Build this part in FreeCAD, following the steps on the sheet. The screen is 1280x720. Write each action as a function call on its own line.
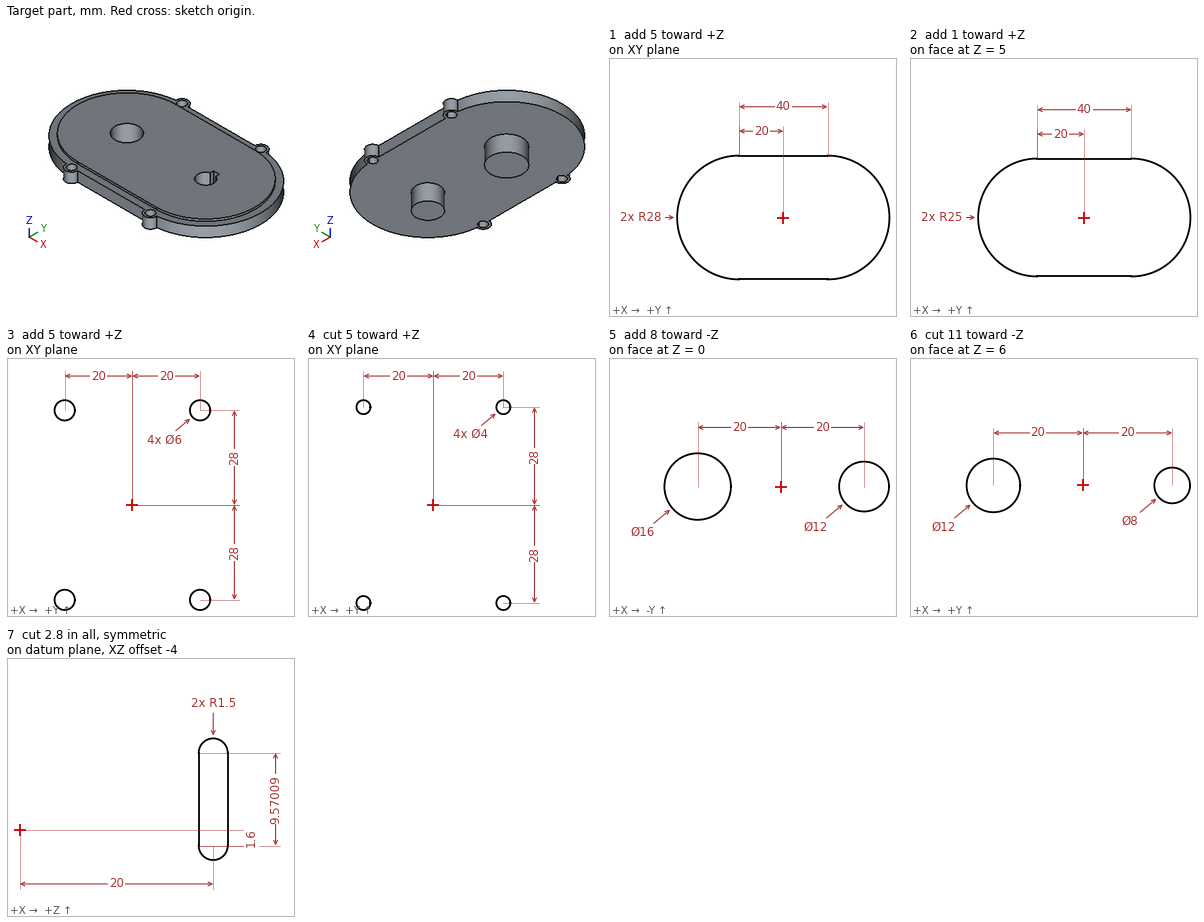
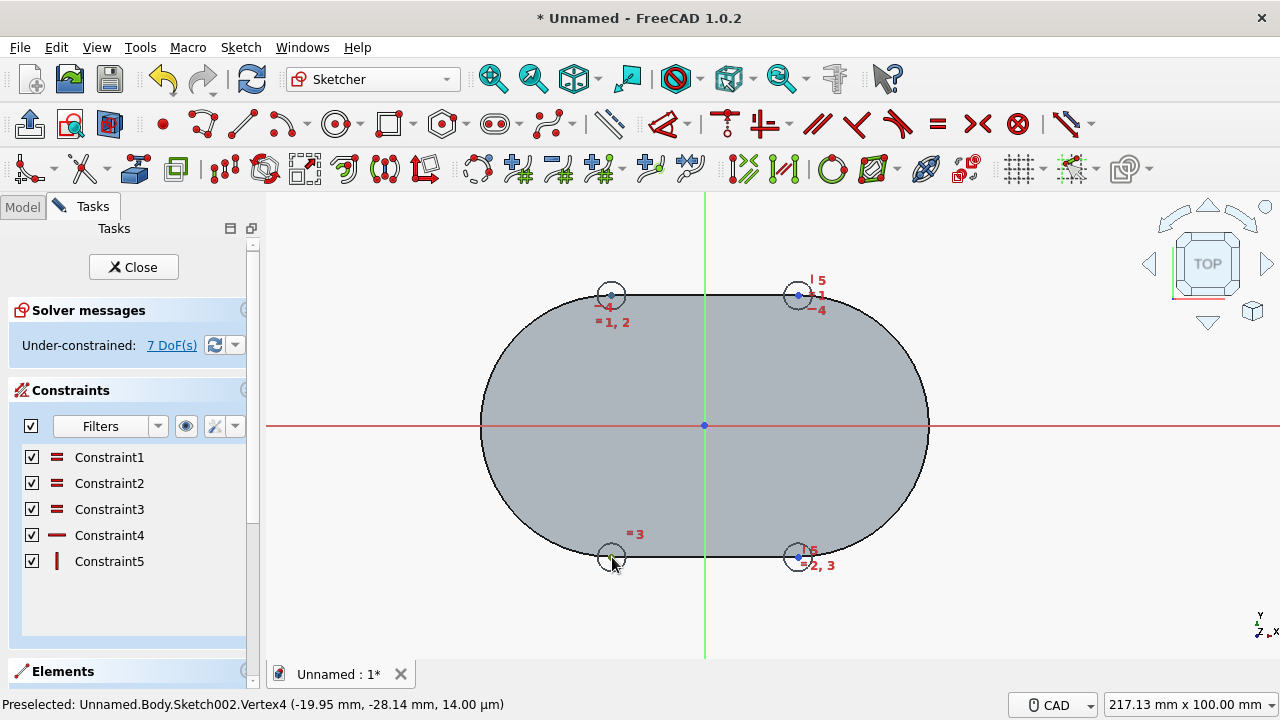
key(v)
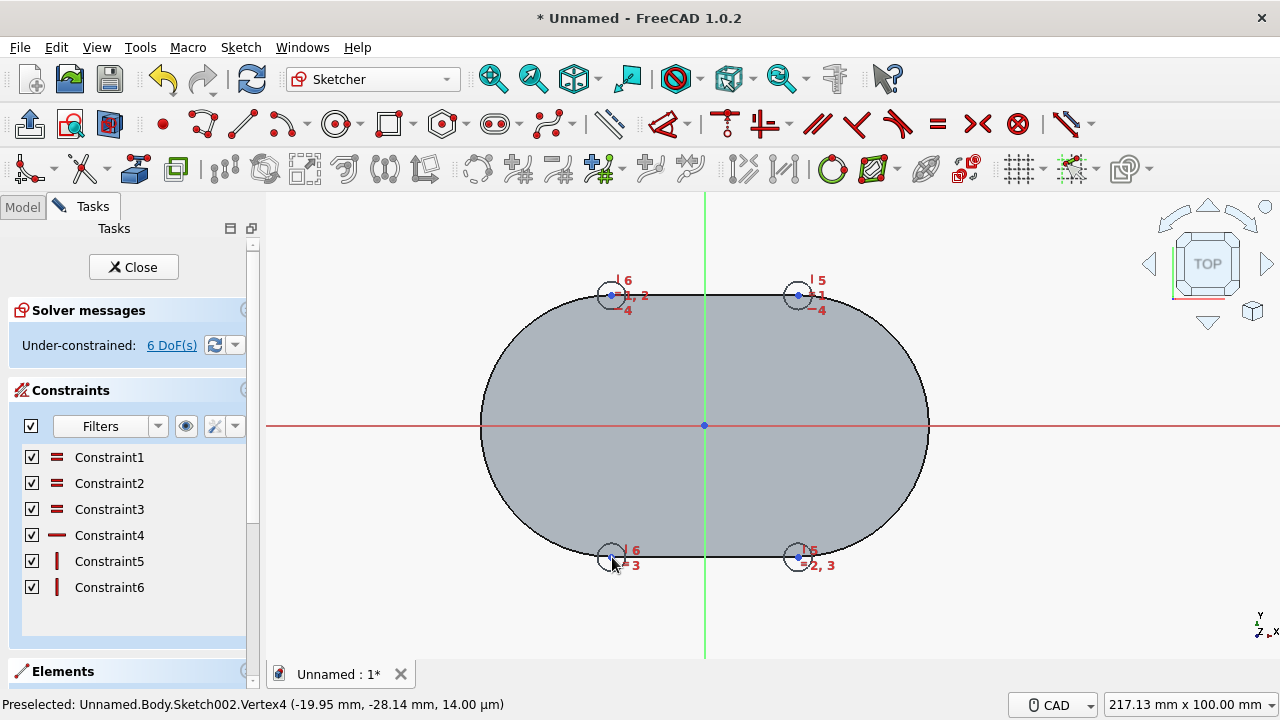
click(798, 557)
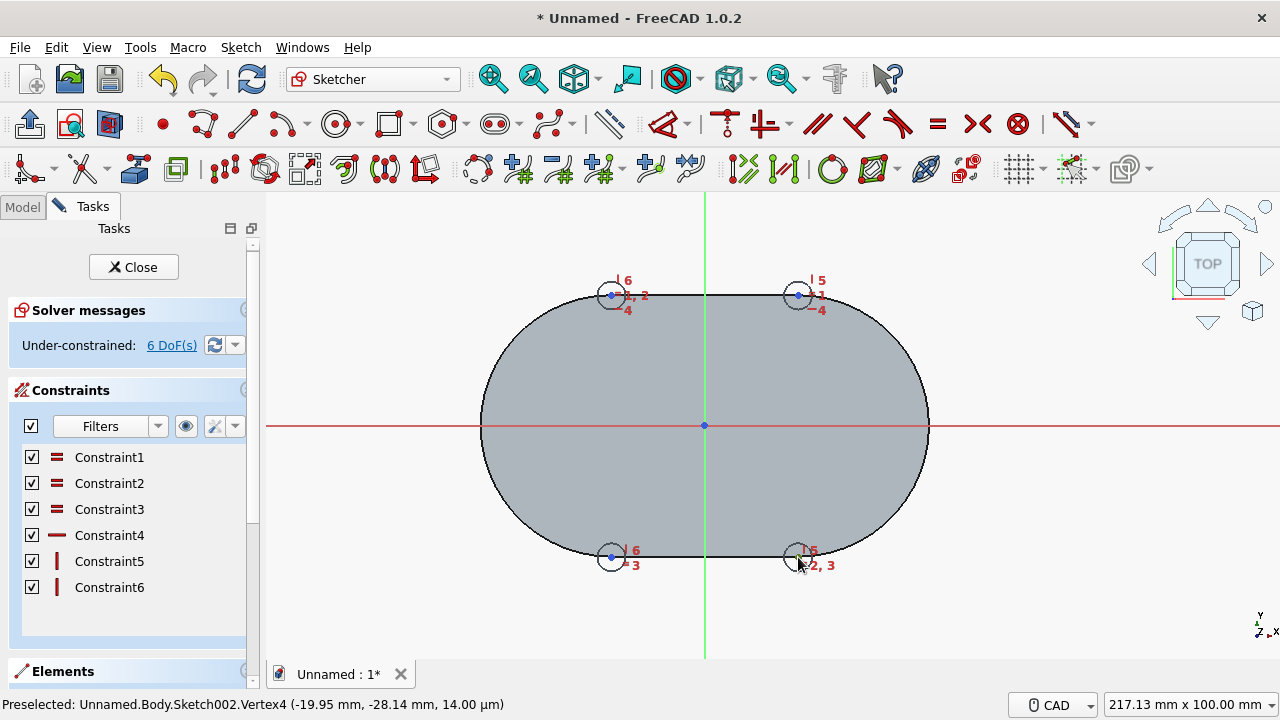
click(611, 557)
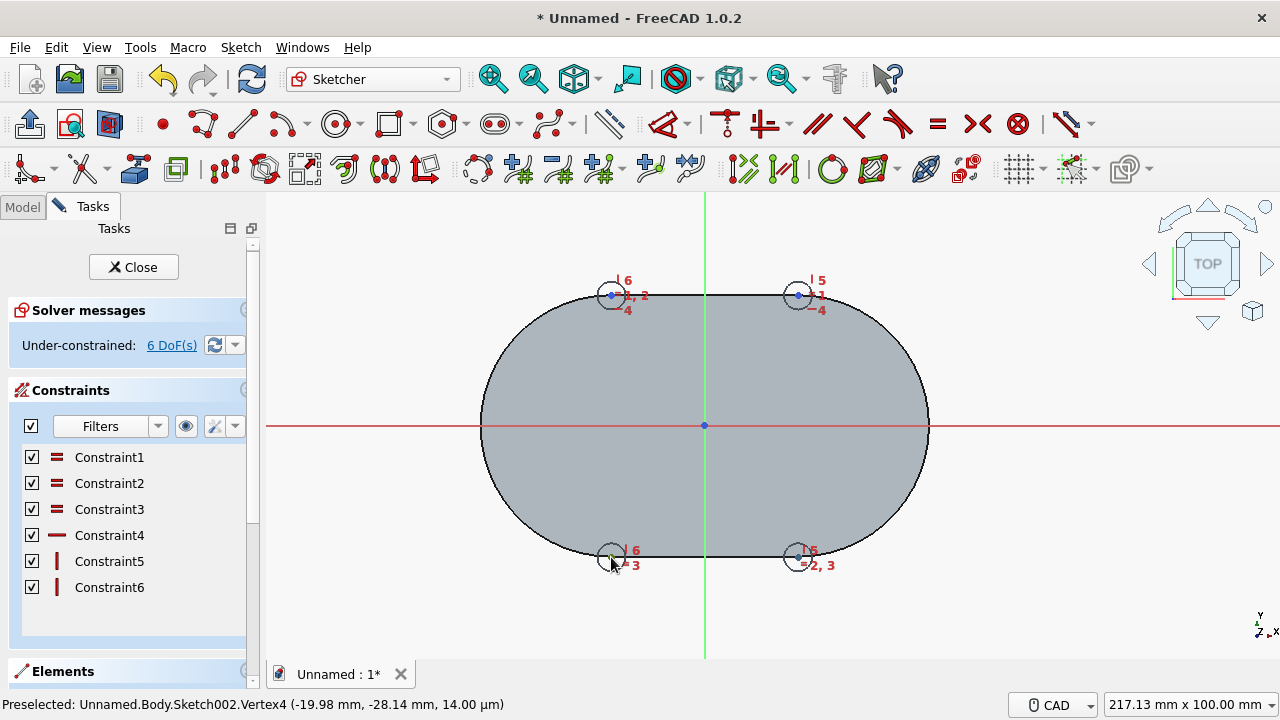
key(h)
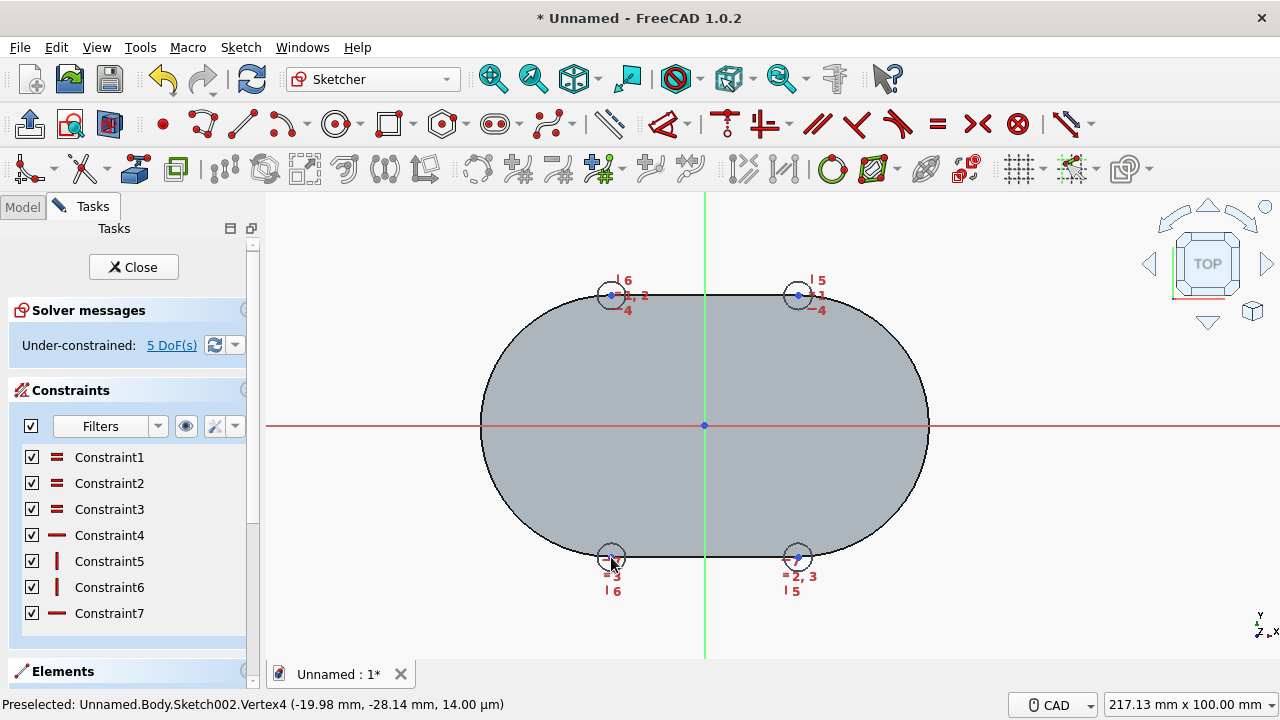
key(d)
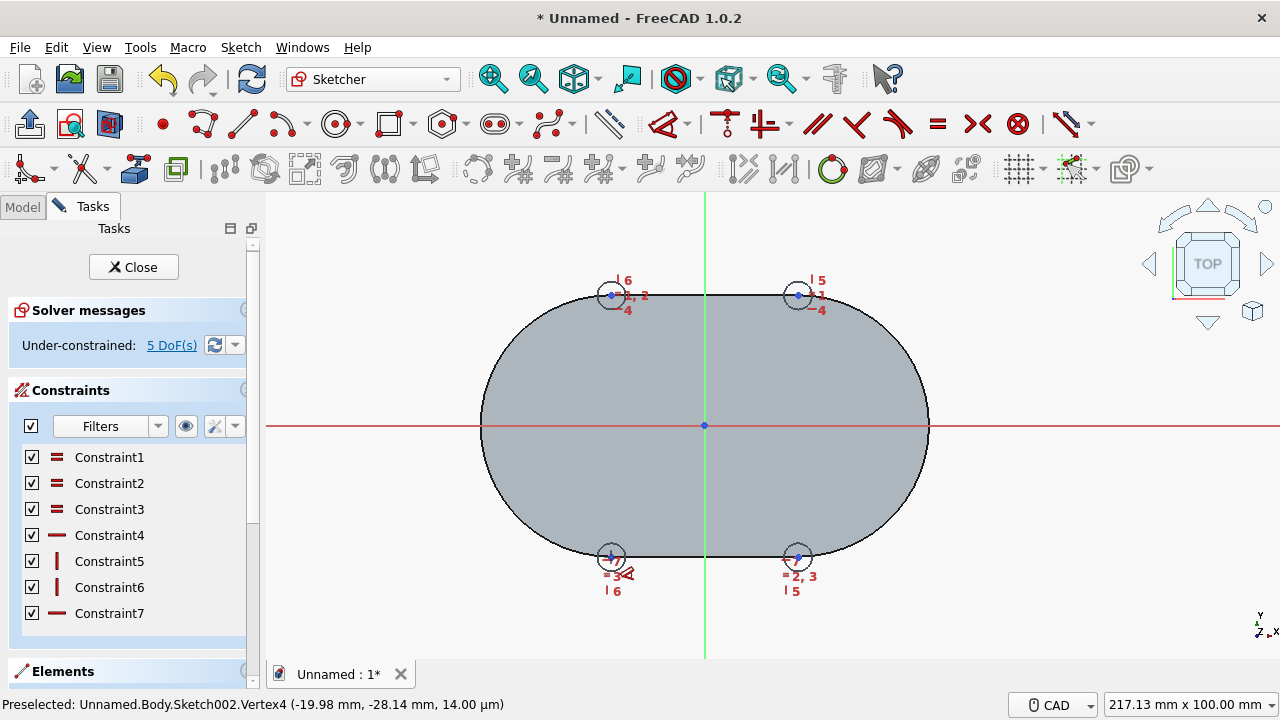
scroll(808, 286, up, 2)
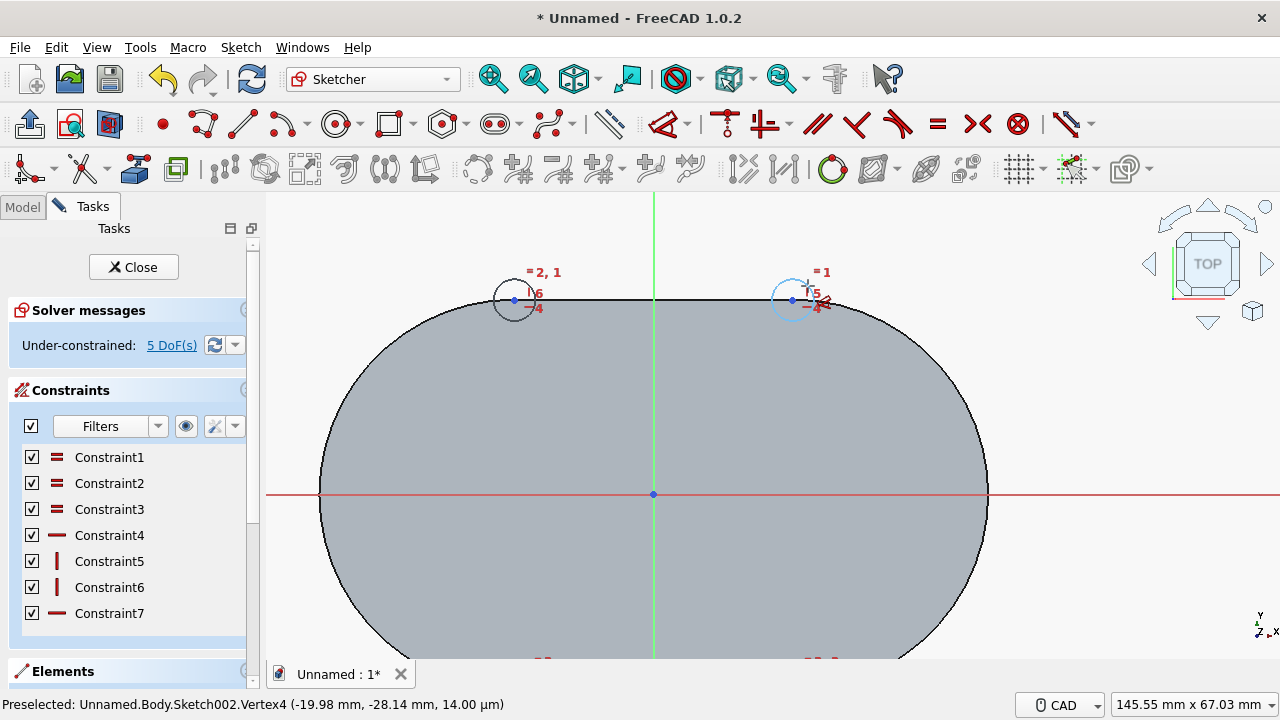
click(808, 285)
click(831, 262)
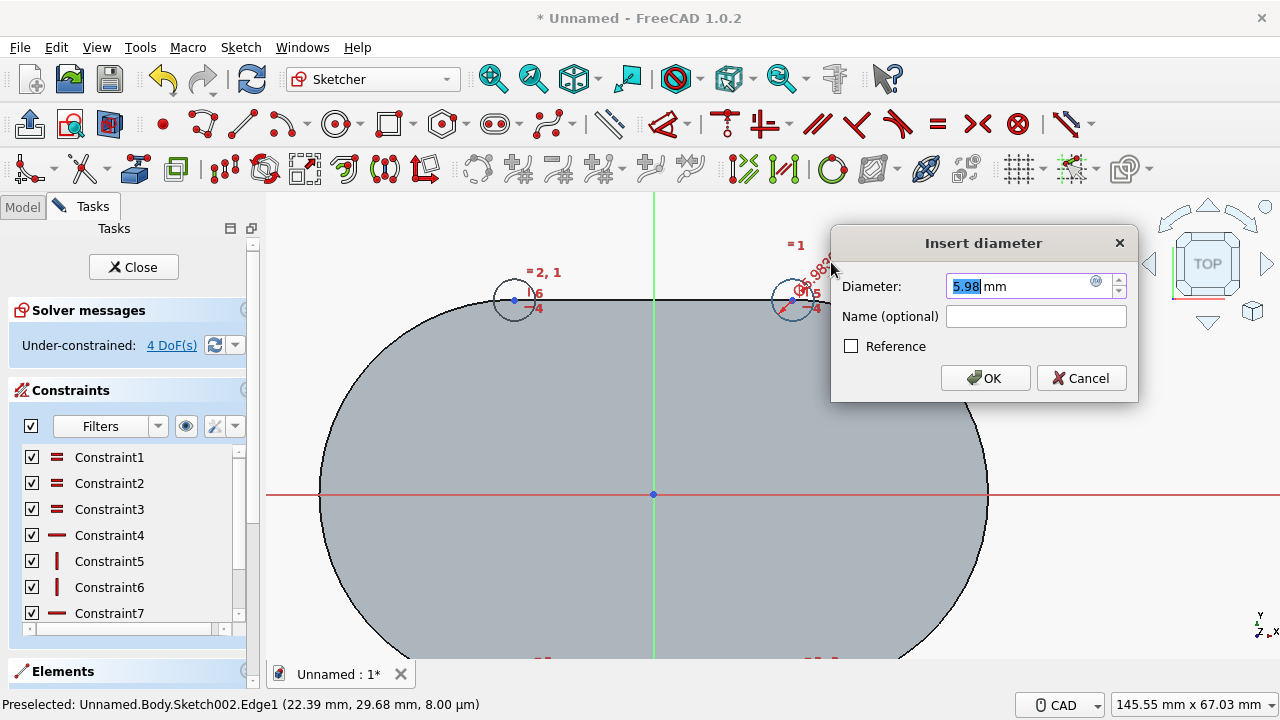
text(6)
key(Return)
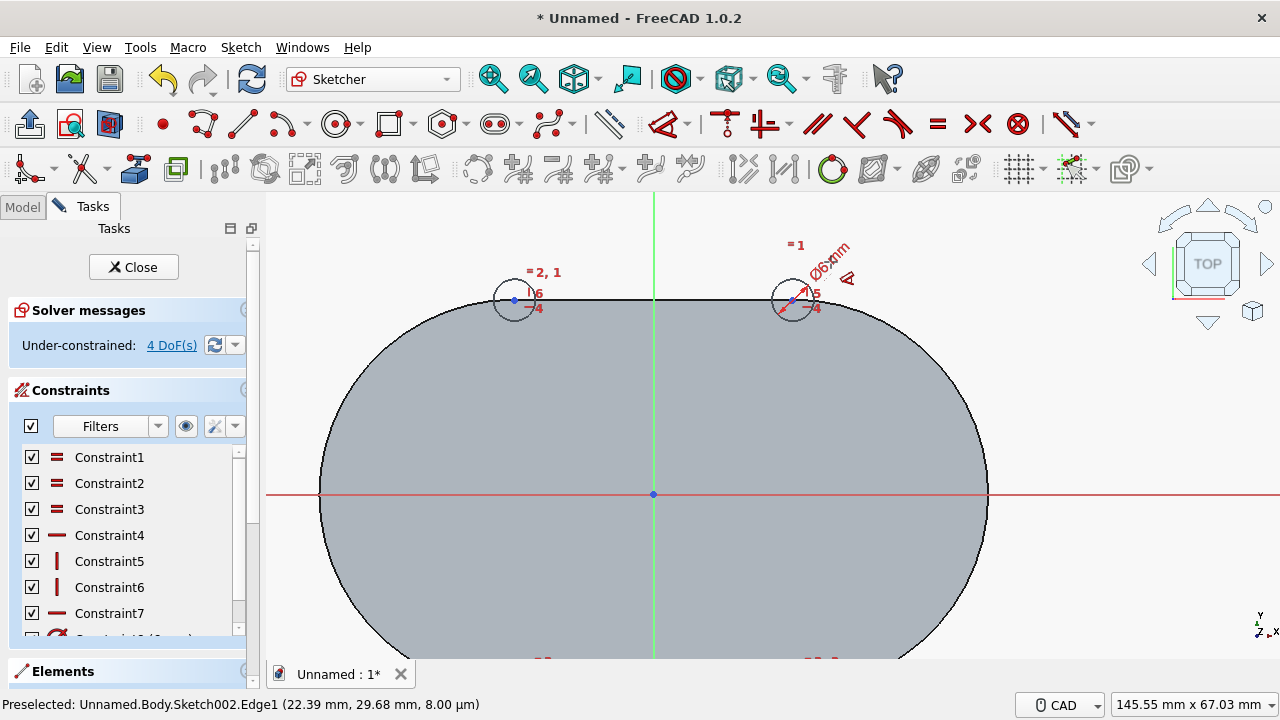
click(793, 300)
click(723, 266)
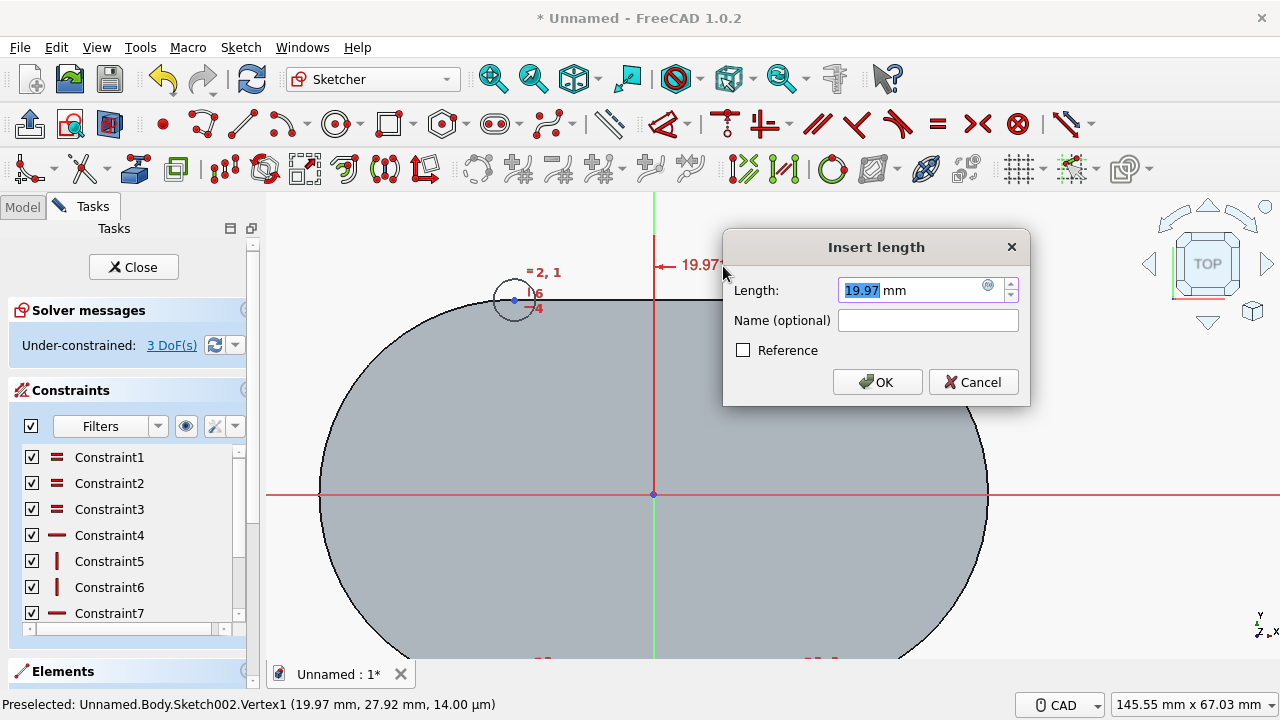
text(20)
key(Return)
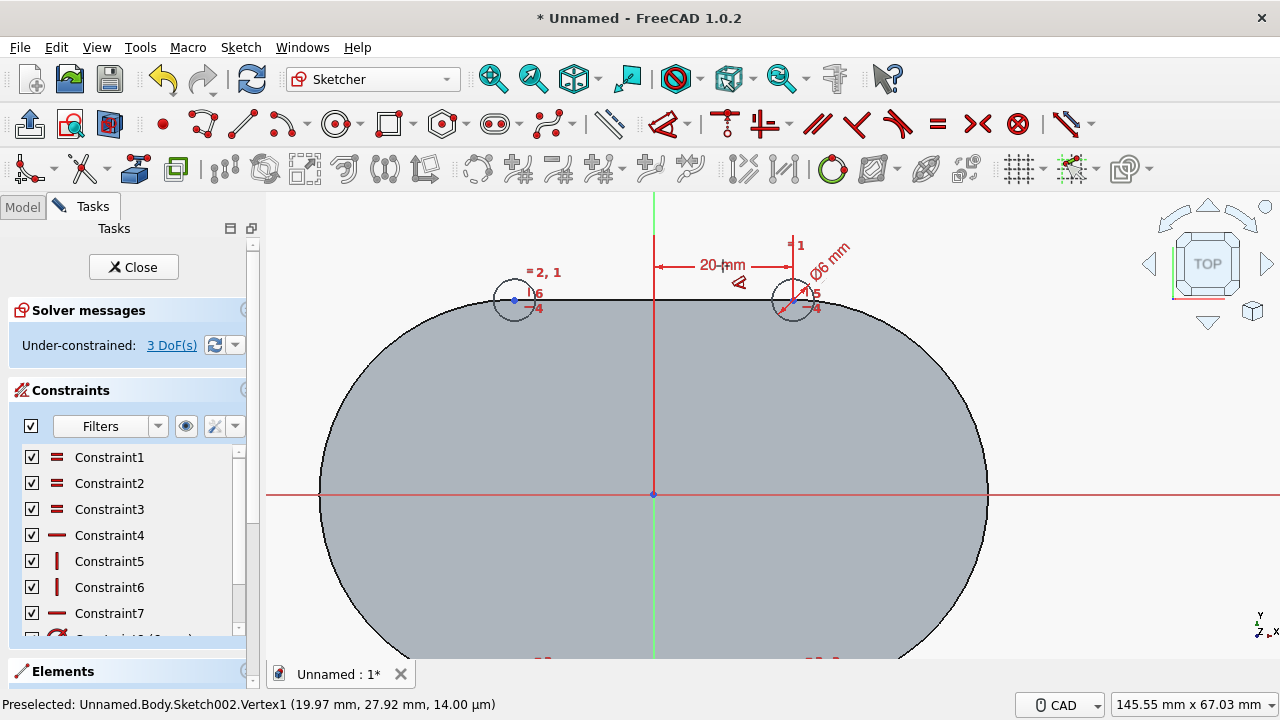
click(793, 300)
click(827, 397)